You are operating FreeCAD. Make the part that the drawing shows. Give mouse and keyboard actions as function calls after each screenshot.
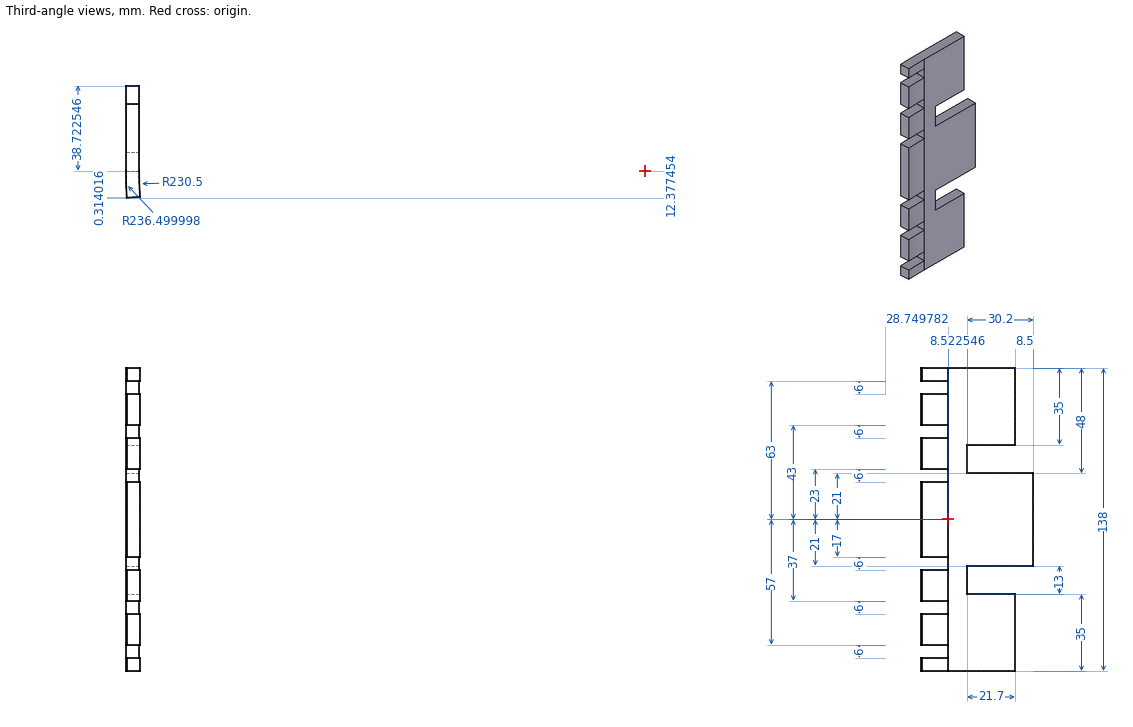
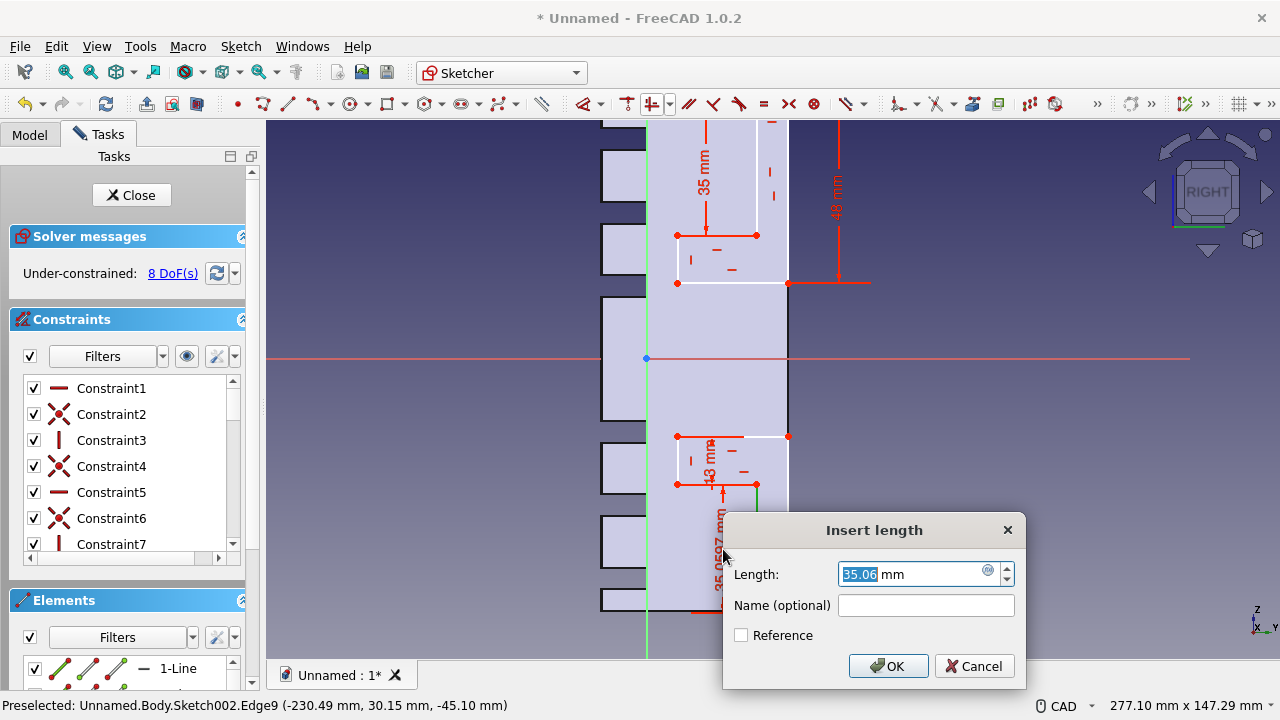
text(35)
key(Return)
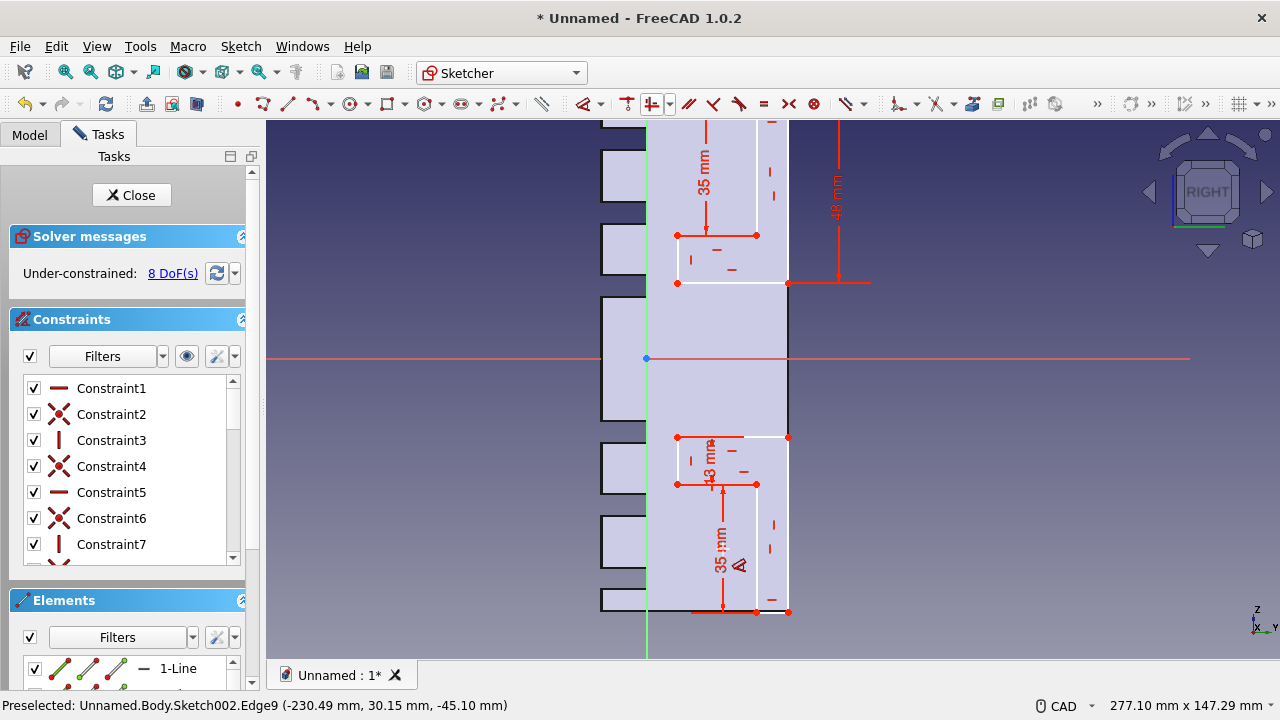
scroll(678, 452, down, 2)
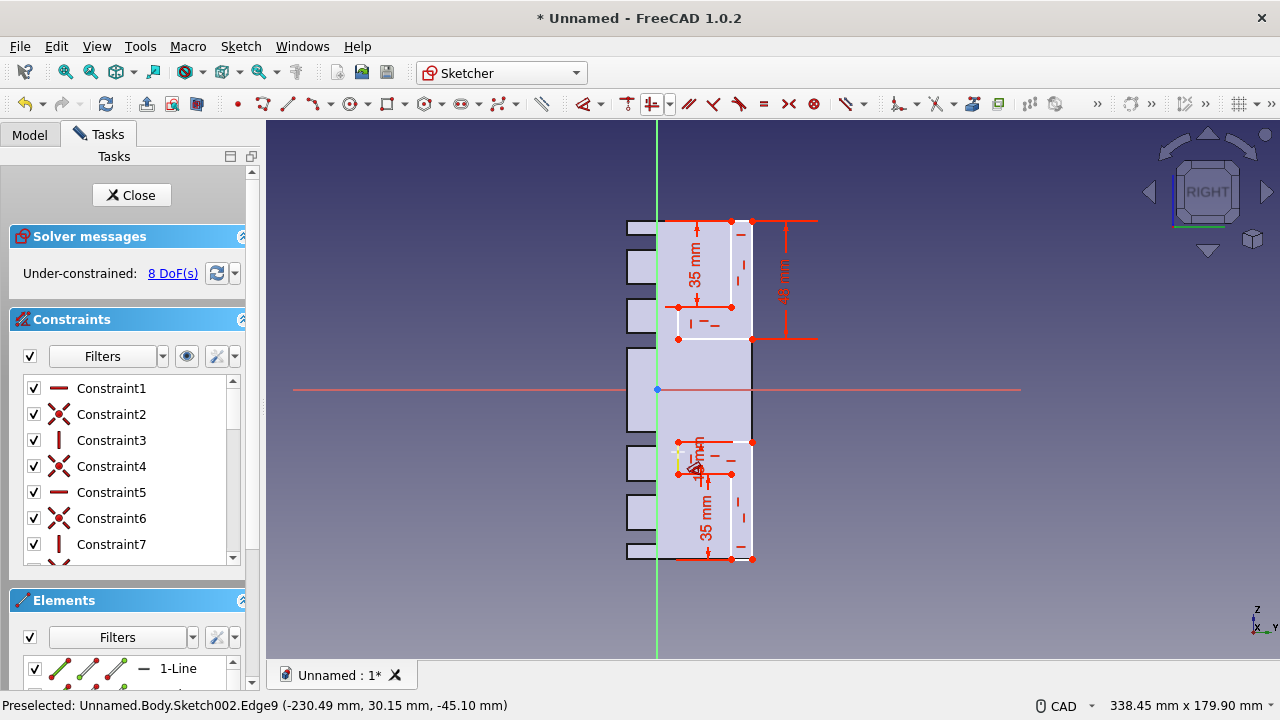
scroll(746, 221, up, 4)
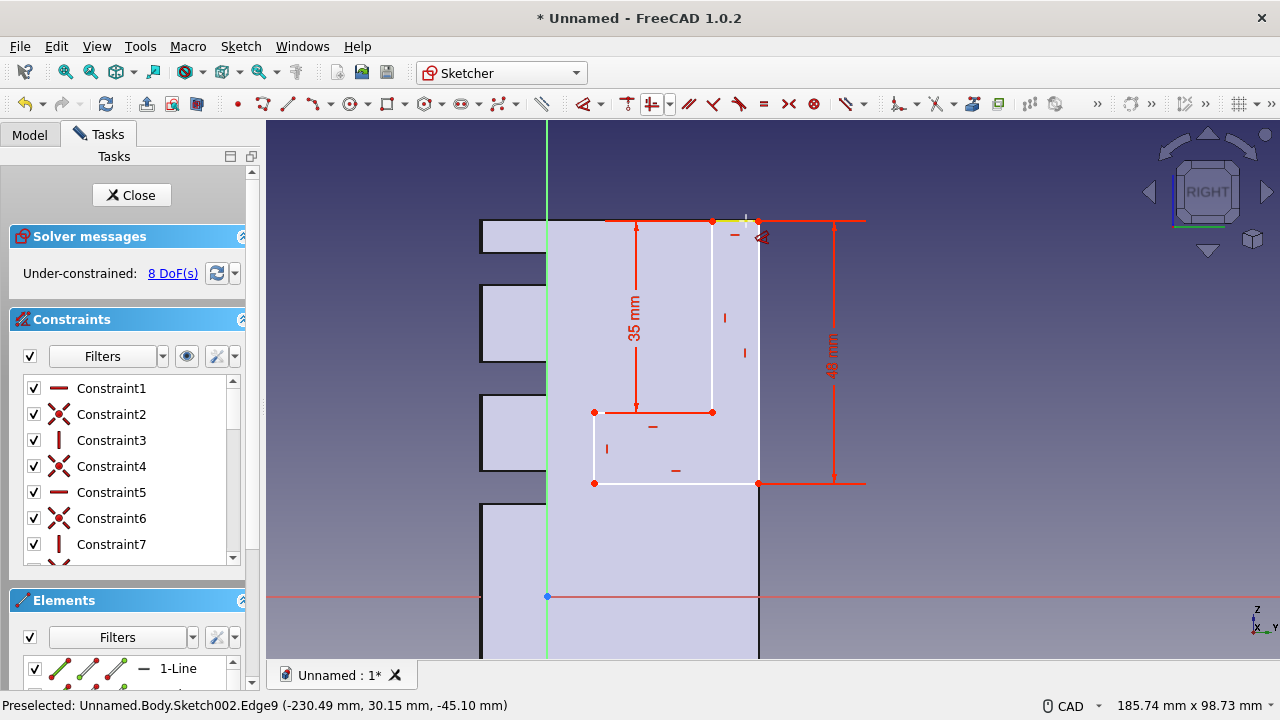
click(745, 221)
click(735, 187)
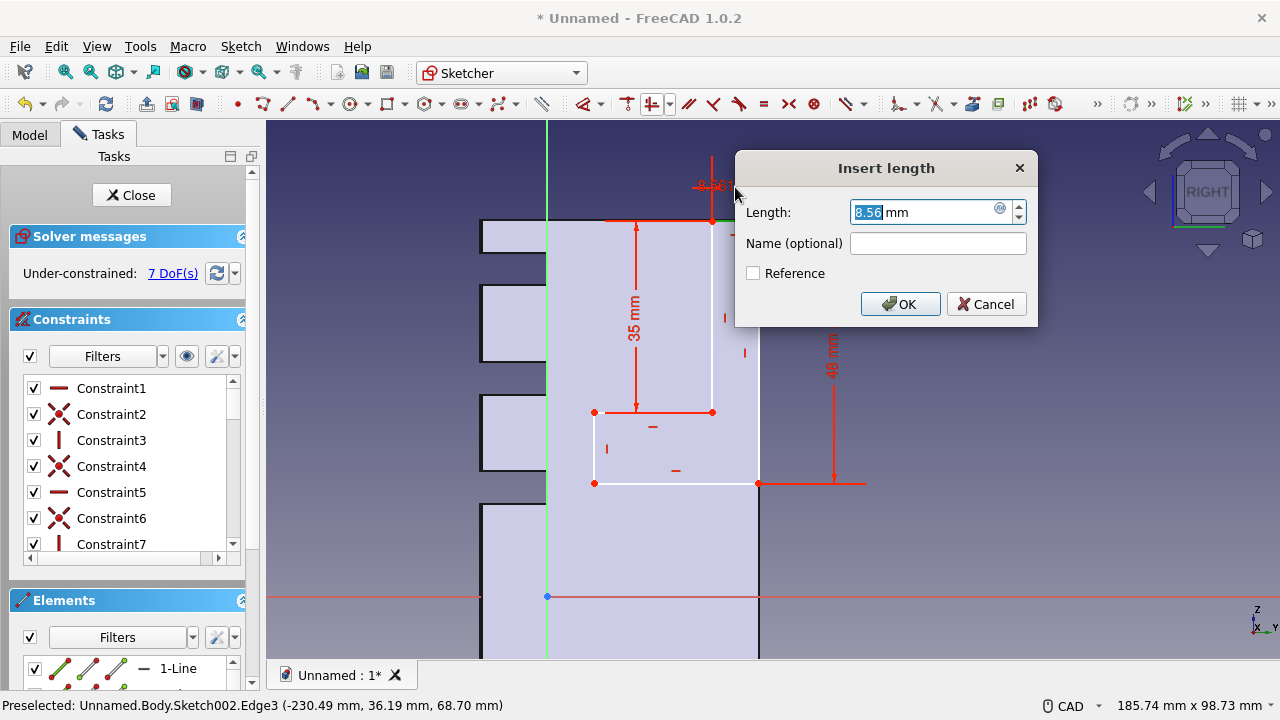
text(8.5)
key(Return)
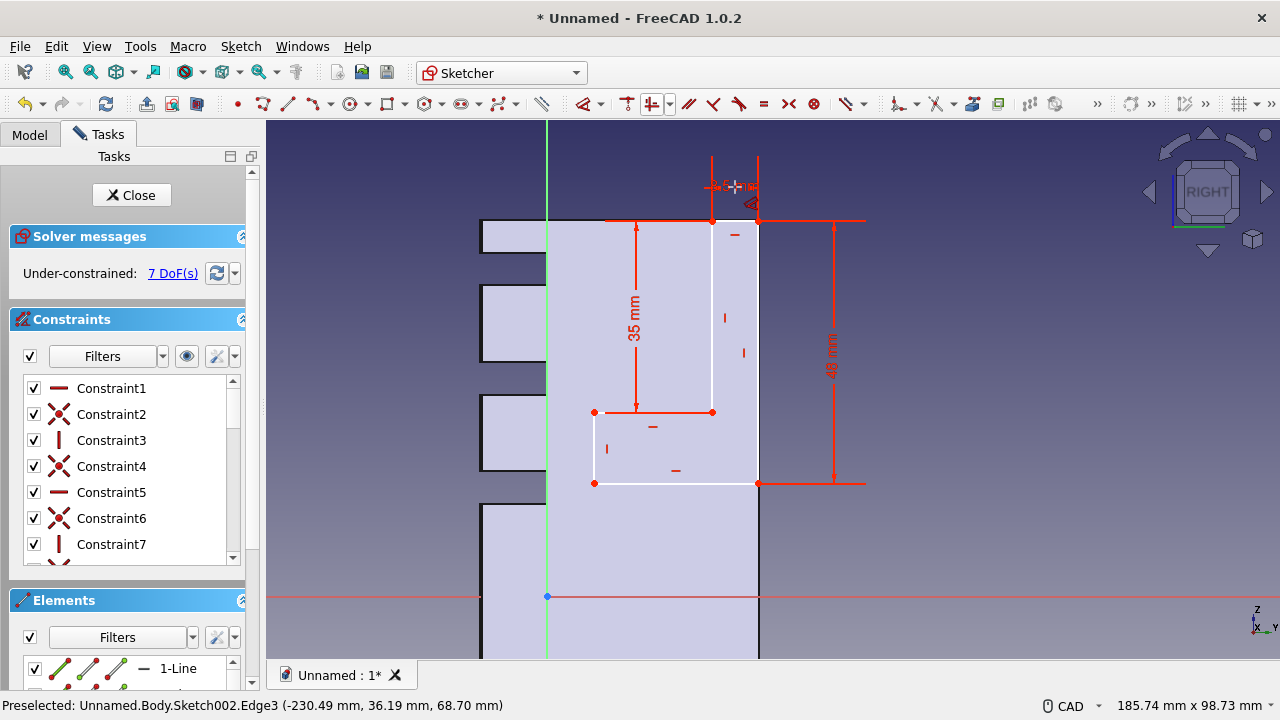
scroll(746, 221, down, 4)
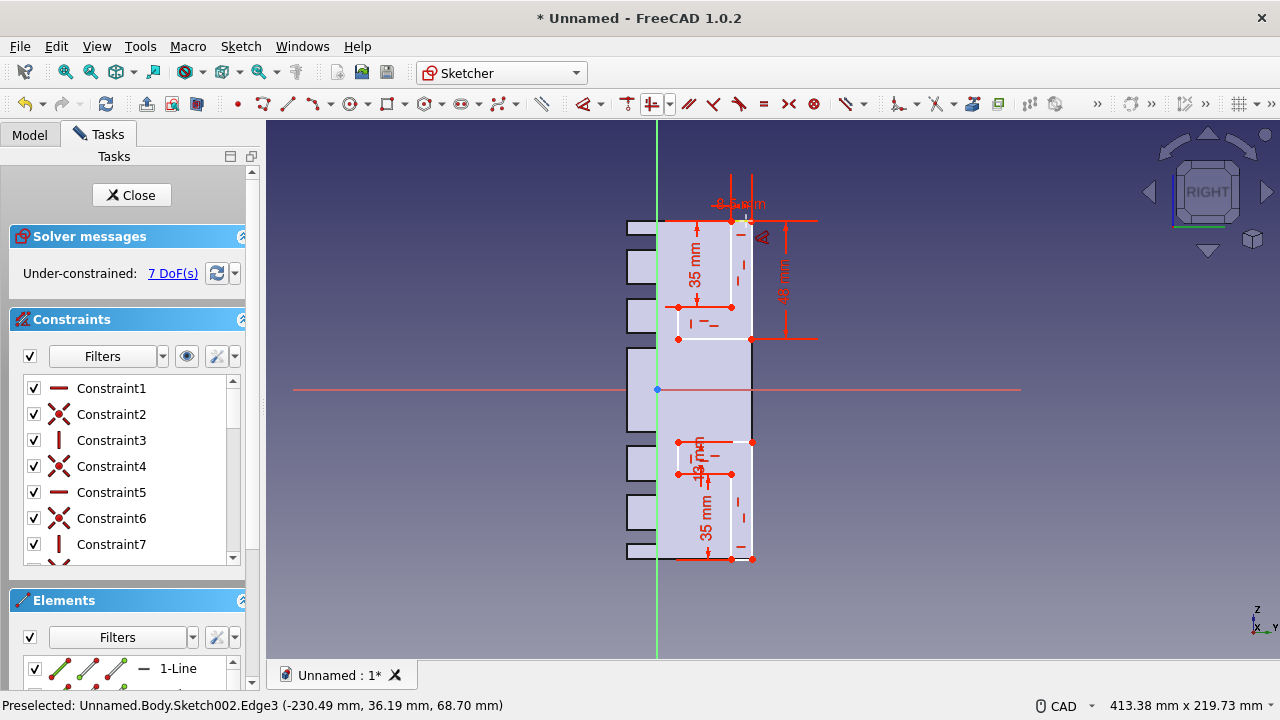
scroll(737, 560, up, 4)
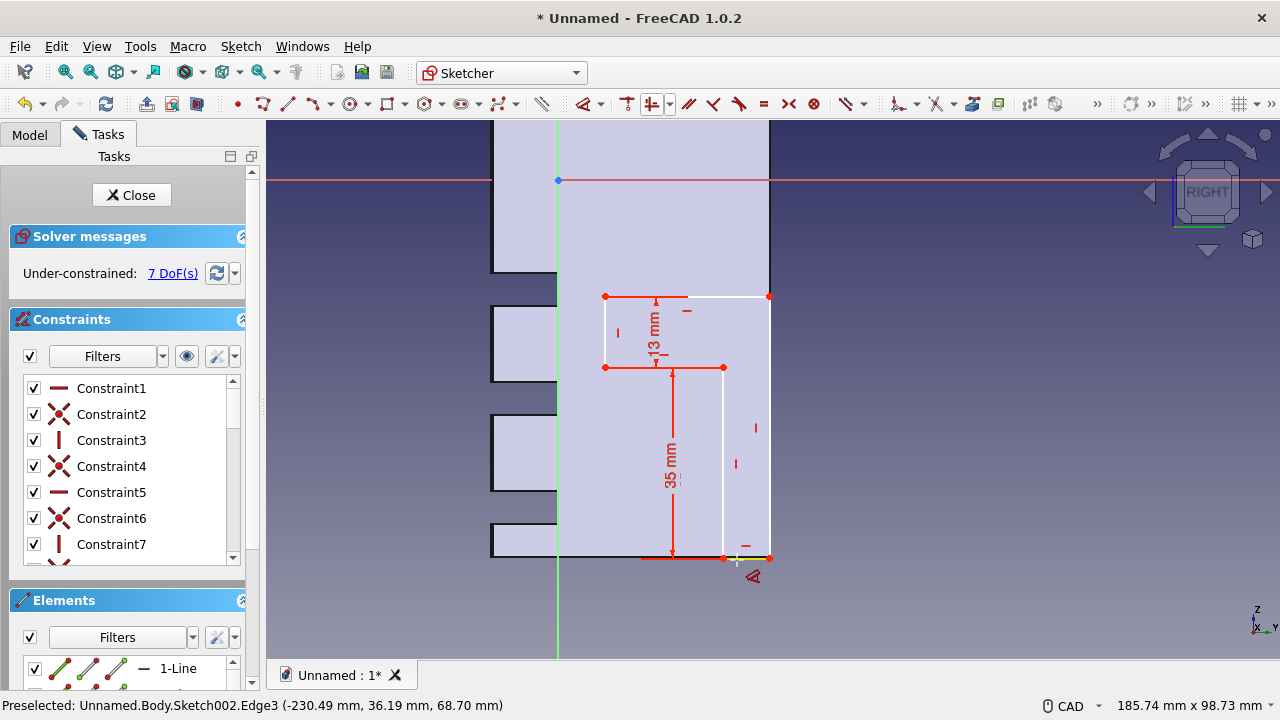
click(737, 559)
click(746, 593)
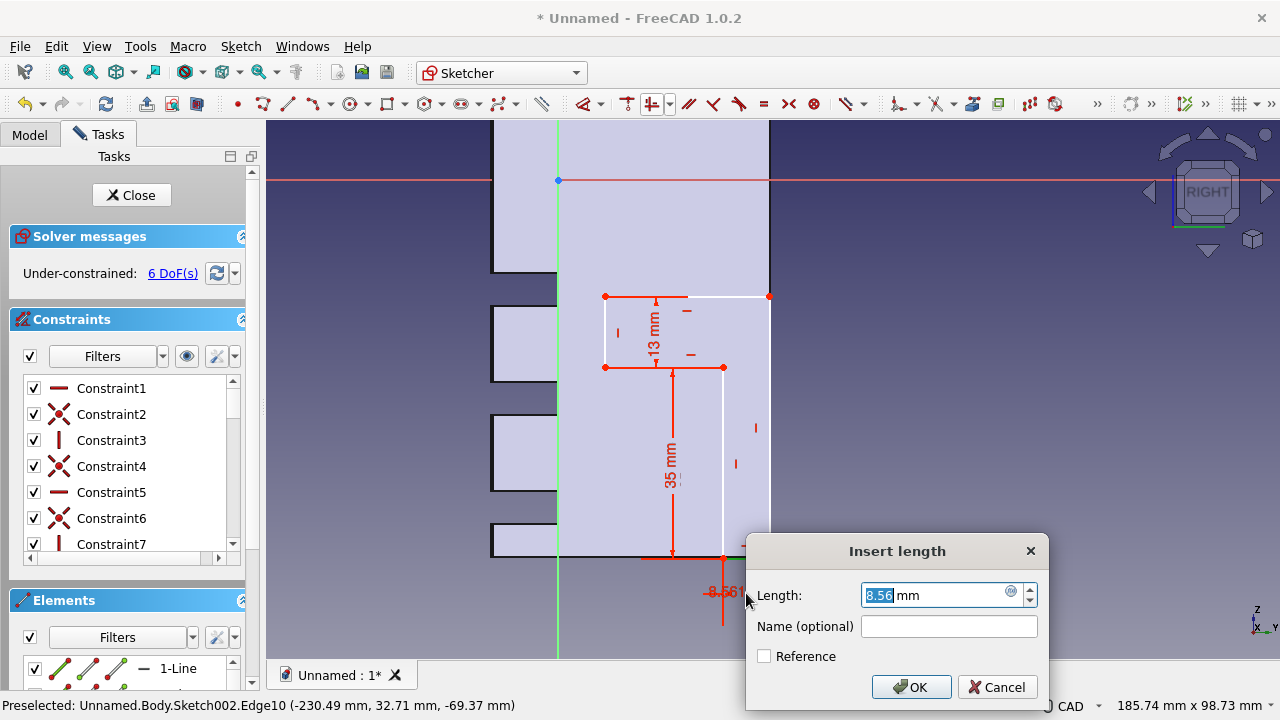
text(8.5)
key(Return)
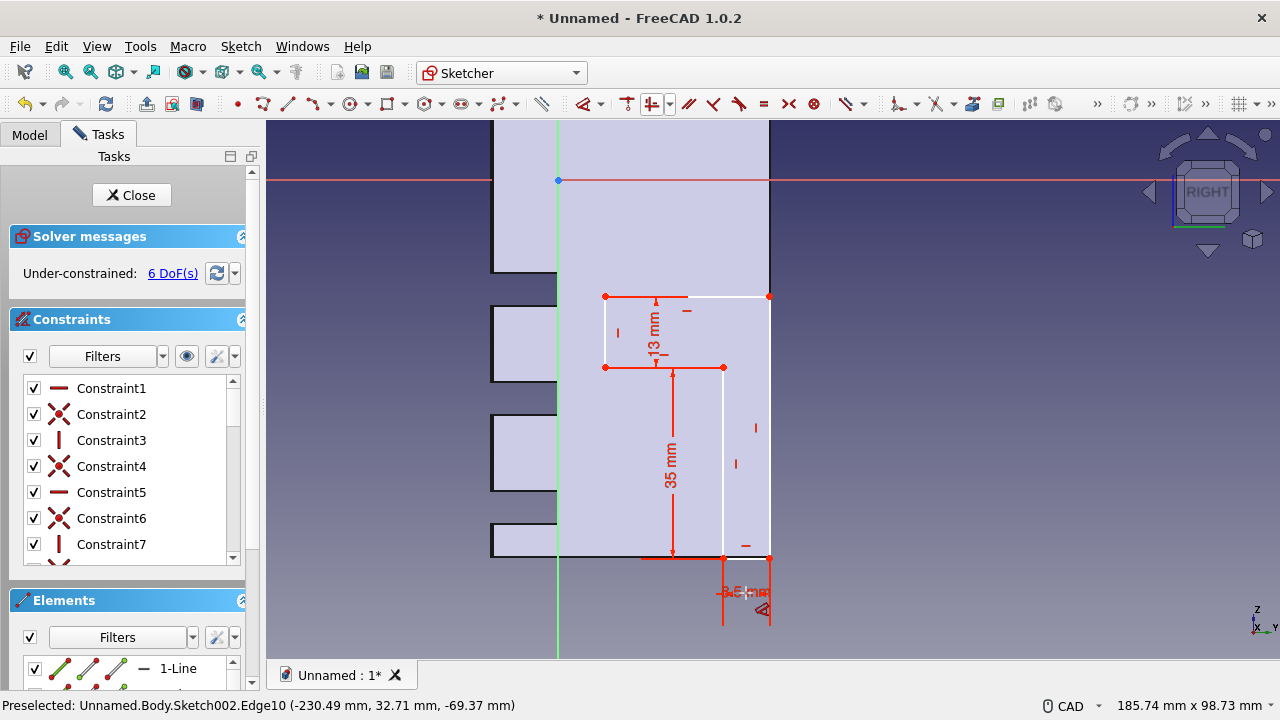
scroll(737, 560, down, 4)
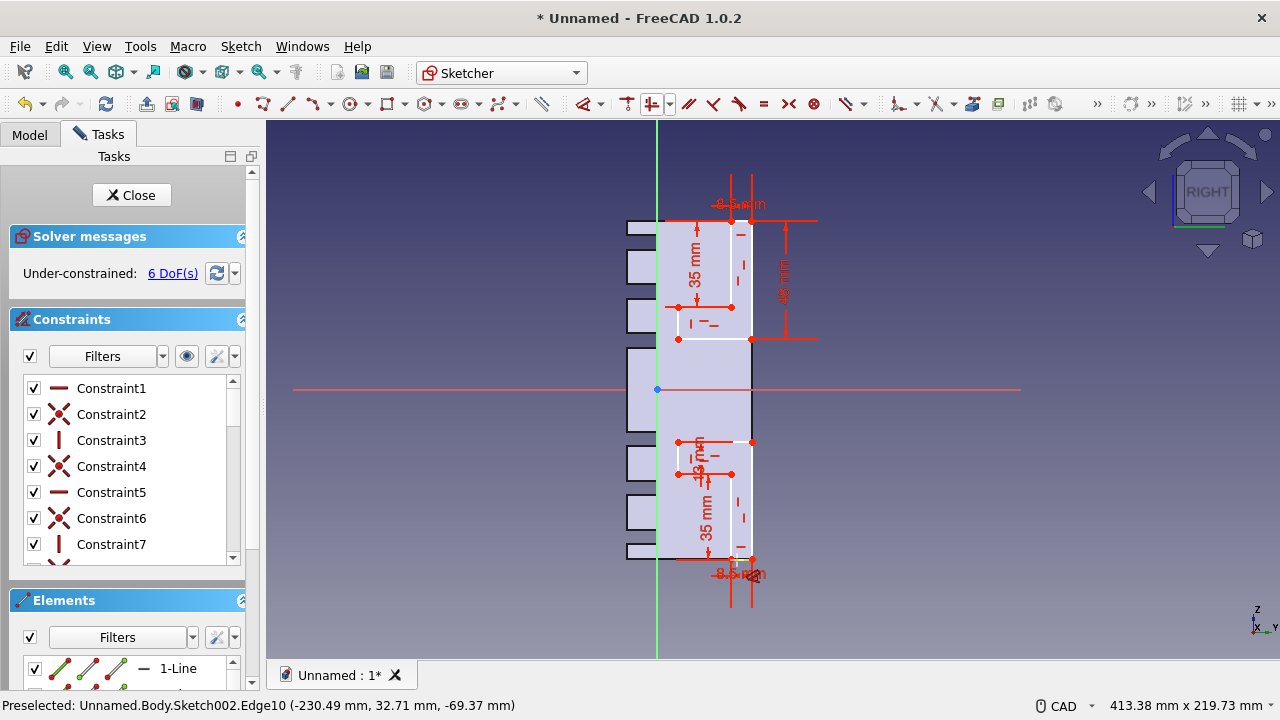
click(678, 339)
click(623, 364)